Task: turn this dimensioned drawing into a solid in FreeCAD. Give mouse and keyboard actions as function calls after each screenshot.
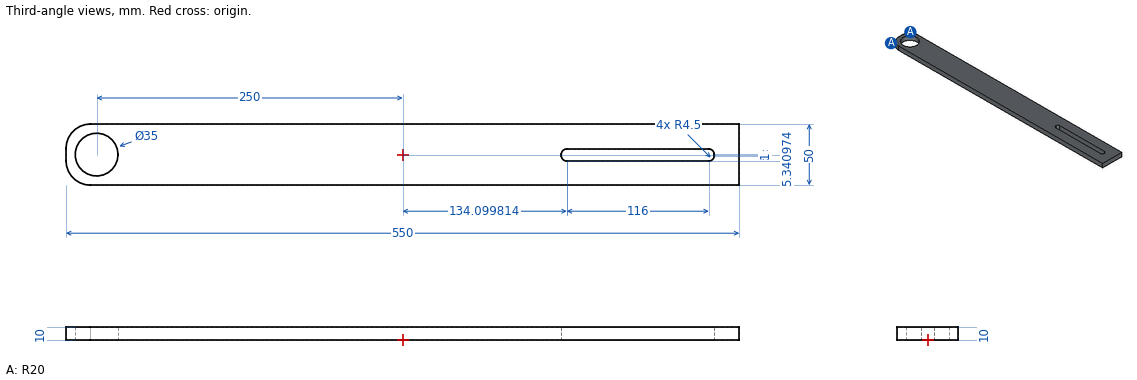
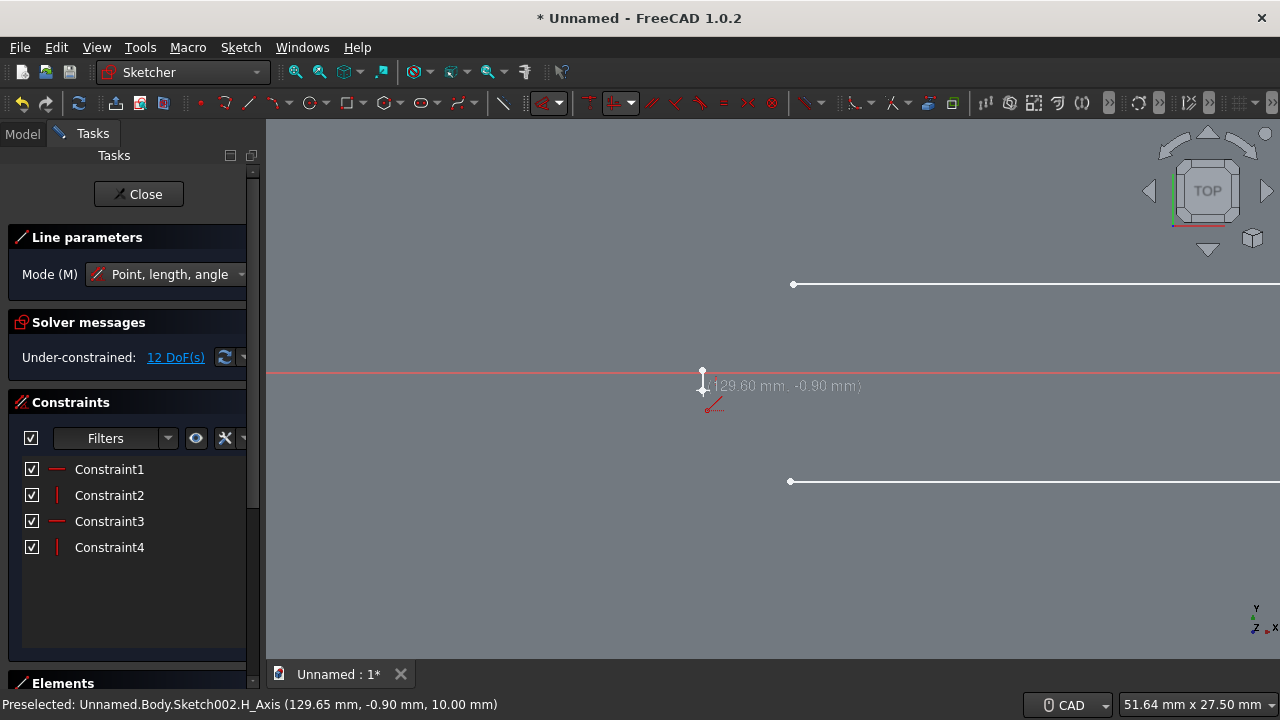
key(g)
key(3)
key(a)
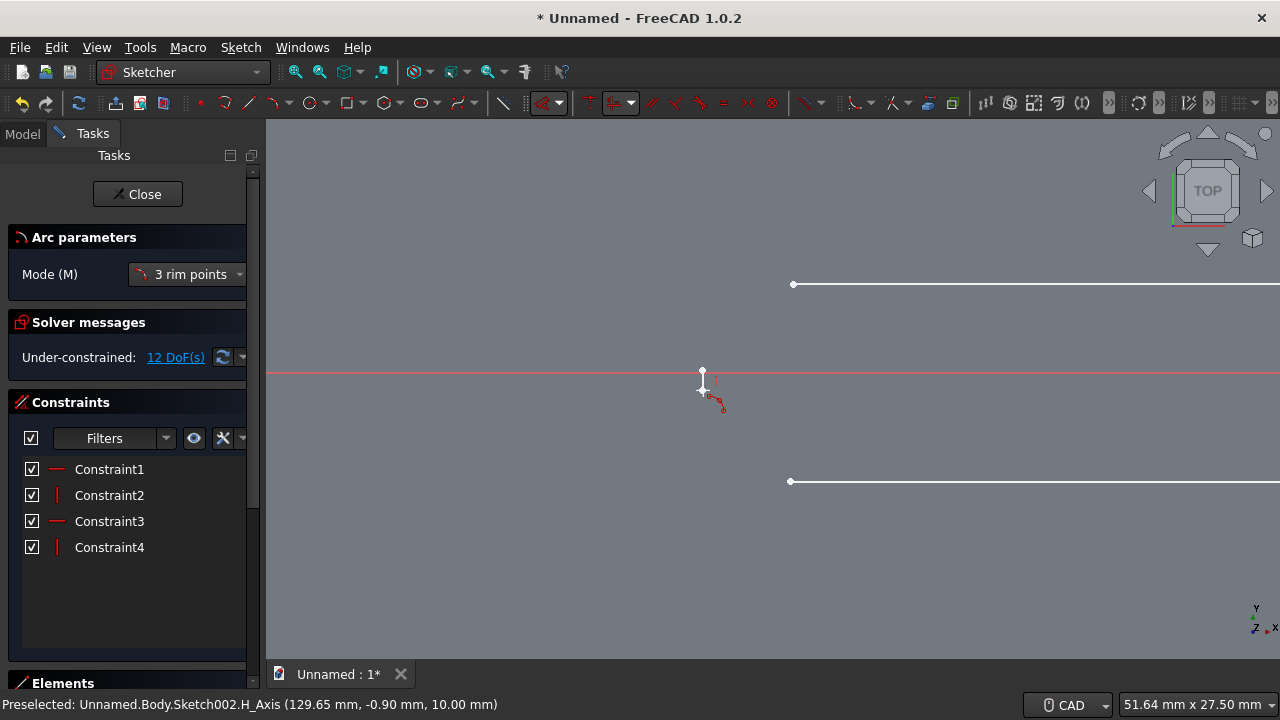
scroll(710, 390, down, 11)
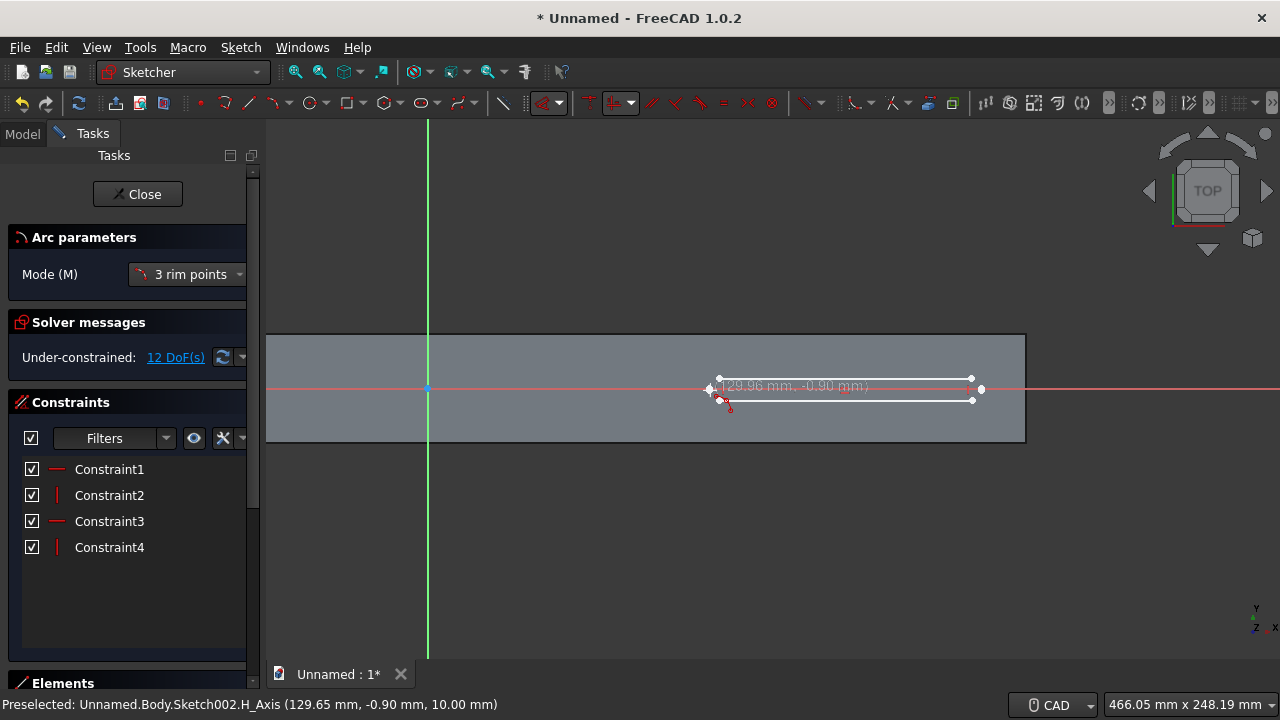
scroll(972, 400, up, 2)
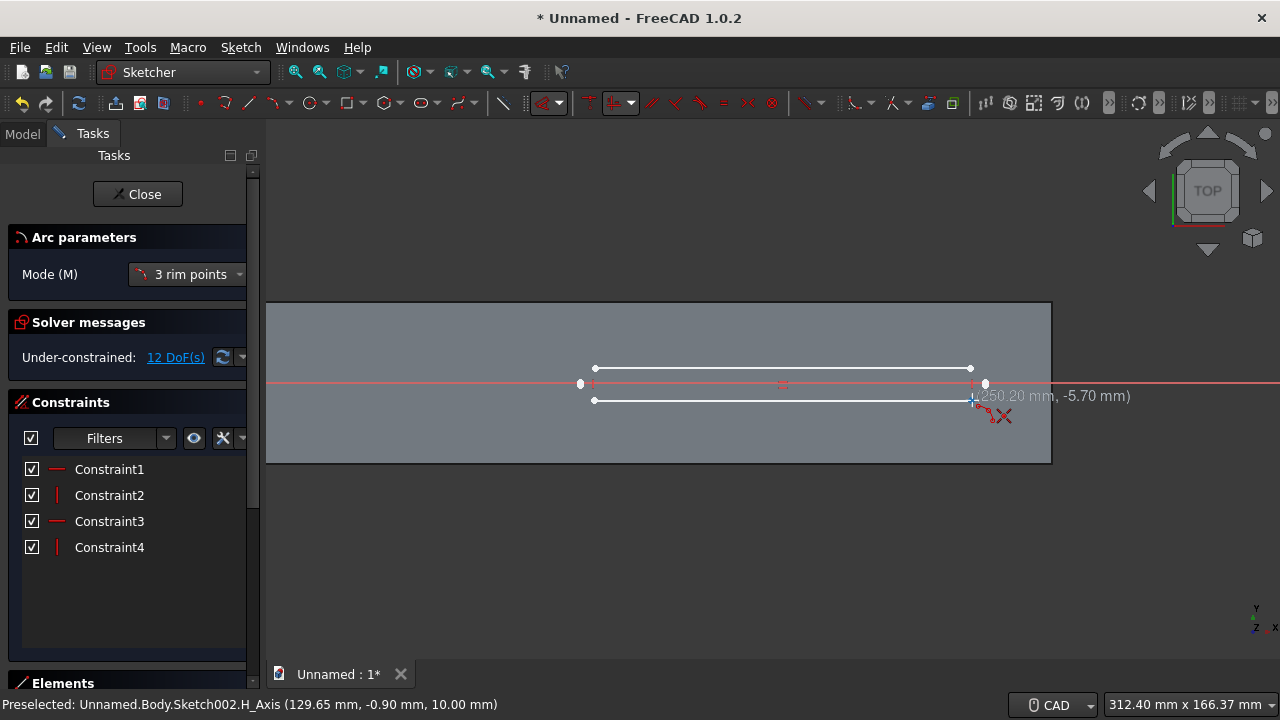
click(972, 401)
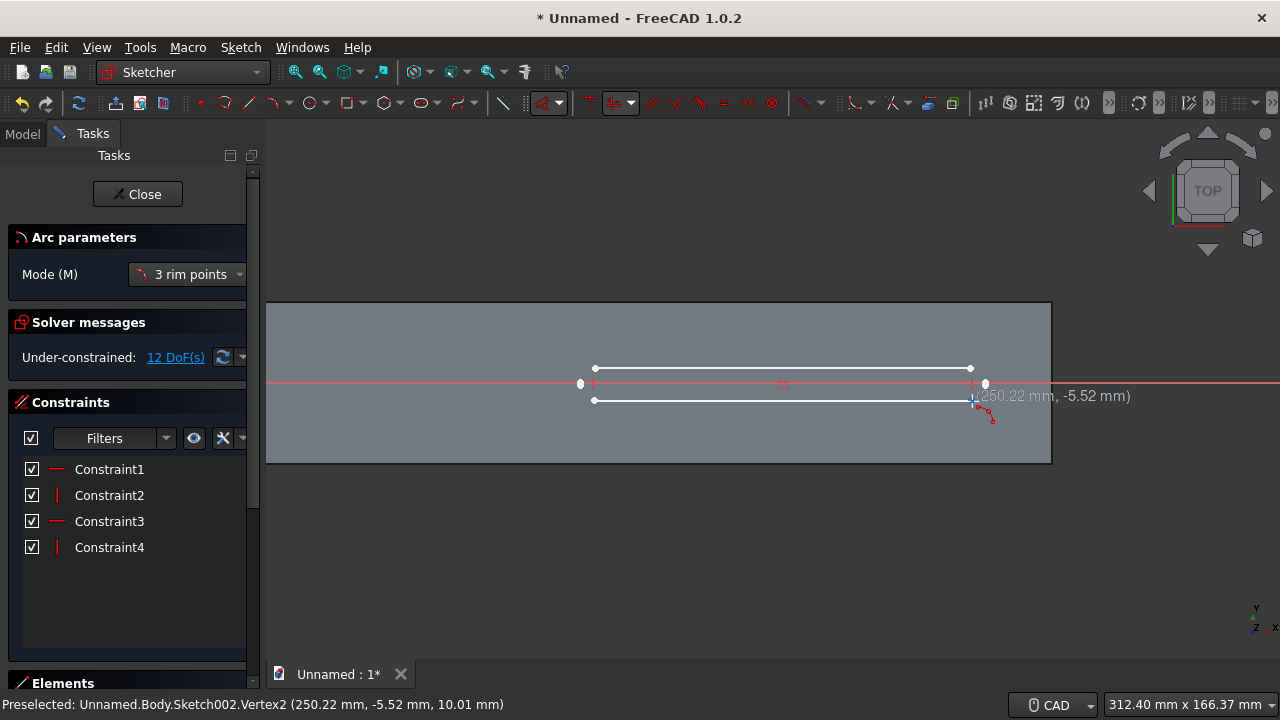
scroll(986, 385, up, 12)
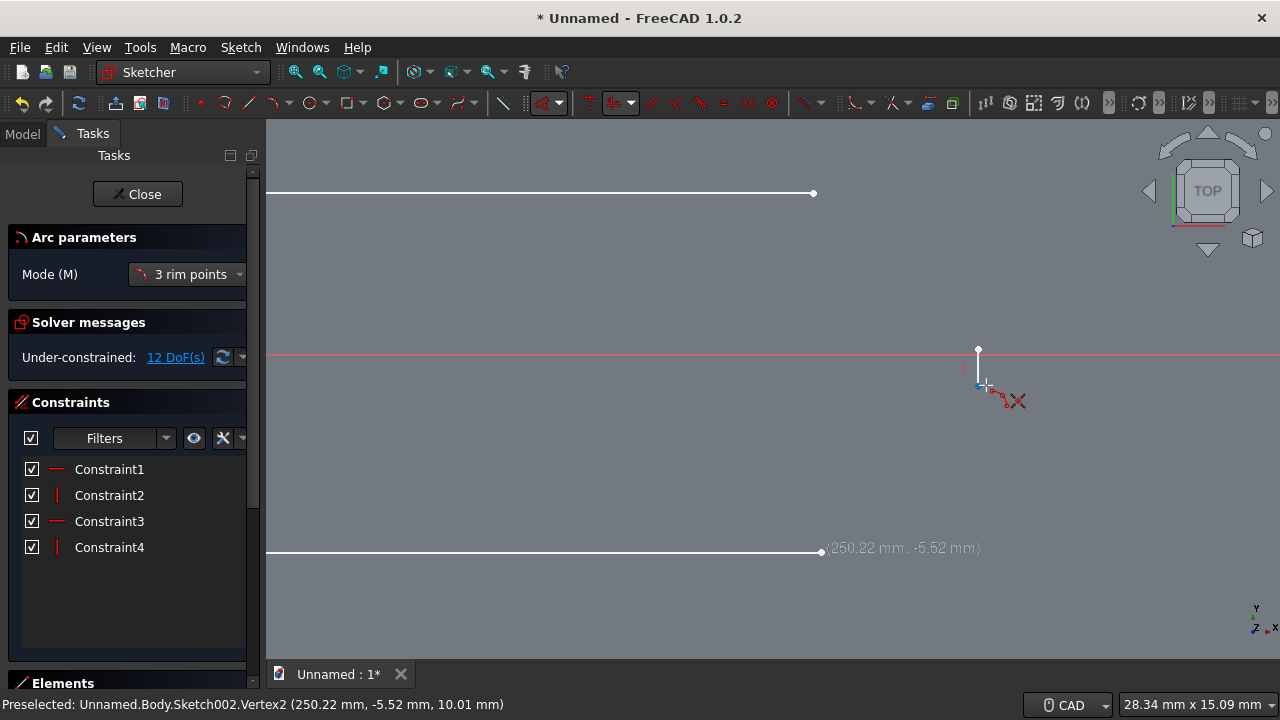
click(978, 386)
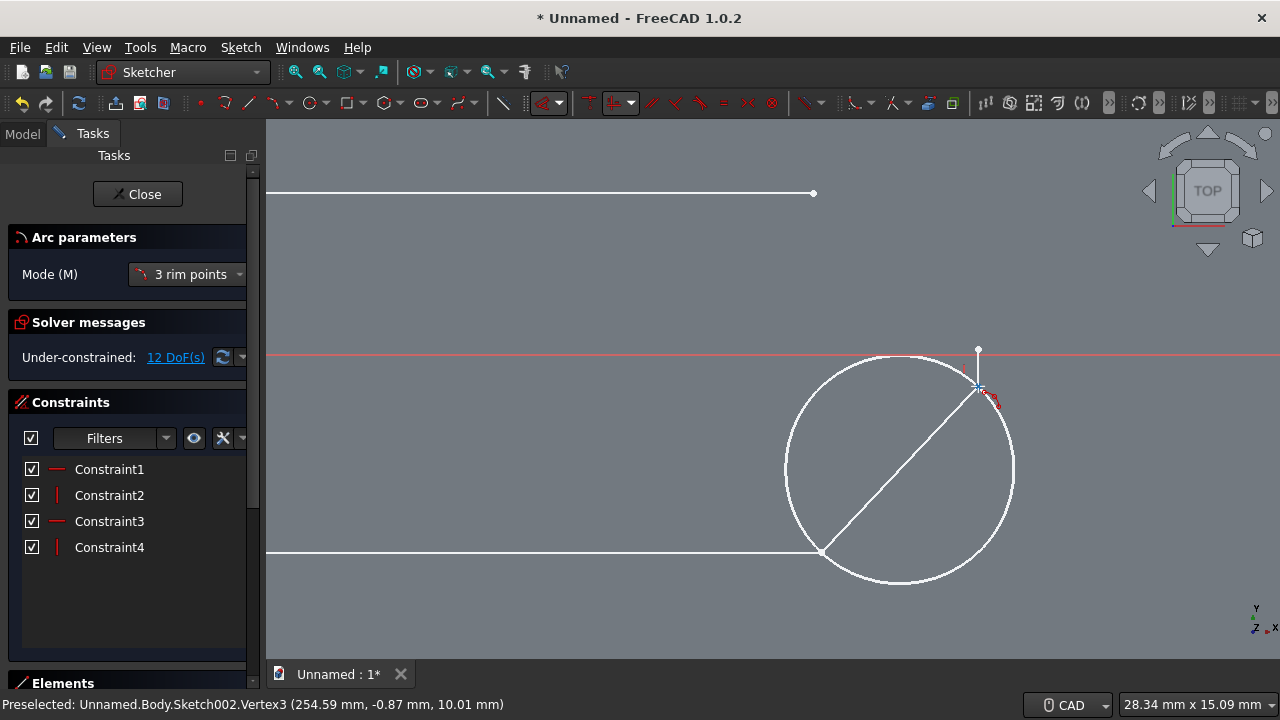
scroll(982, 390, down, 14)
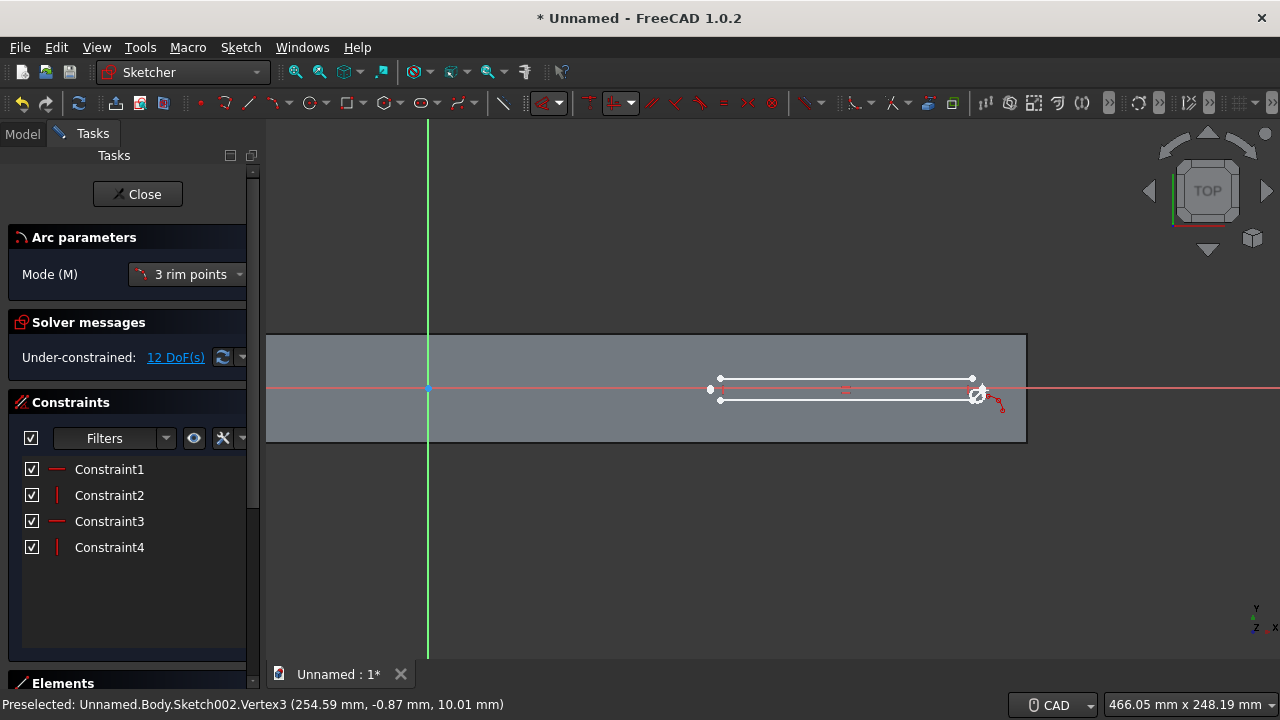
scroll(980, 397, up, 9)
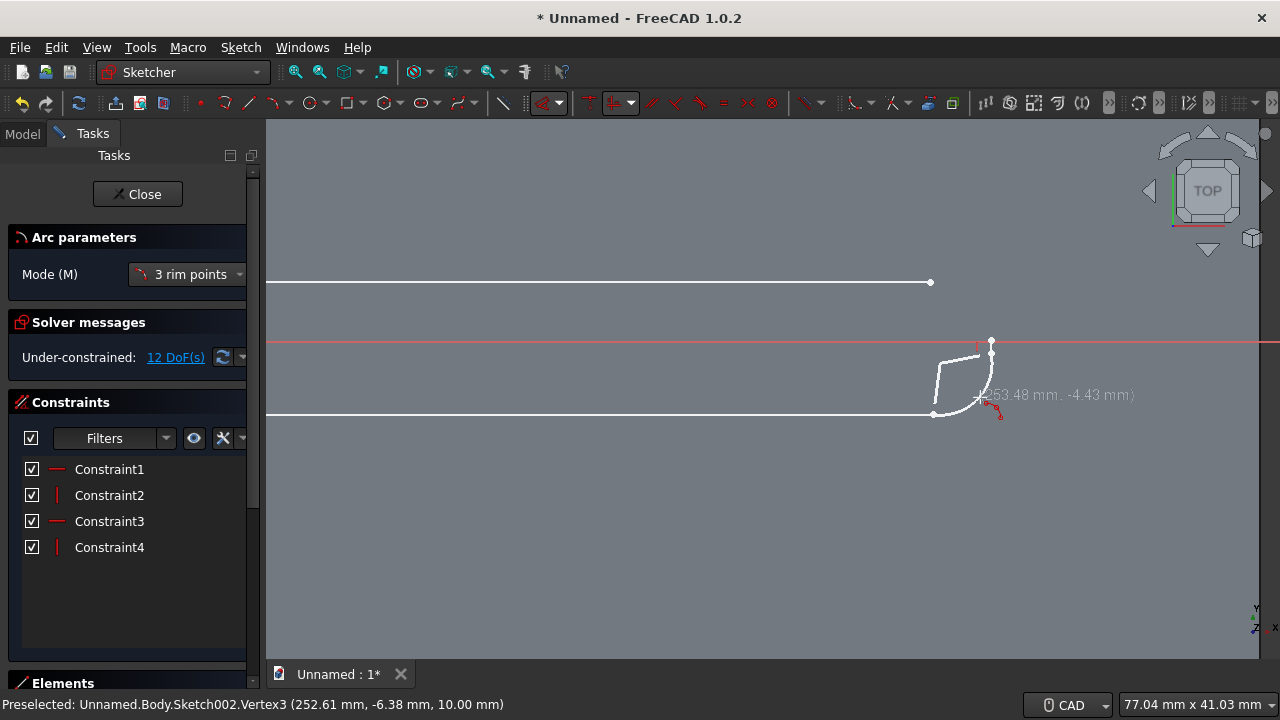
click(974, 395)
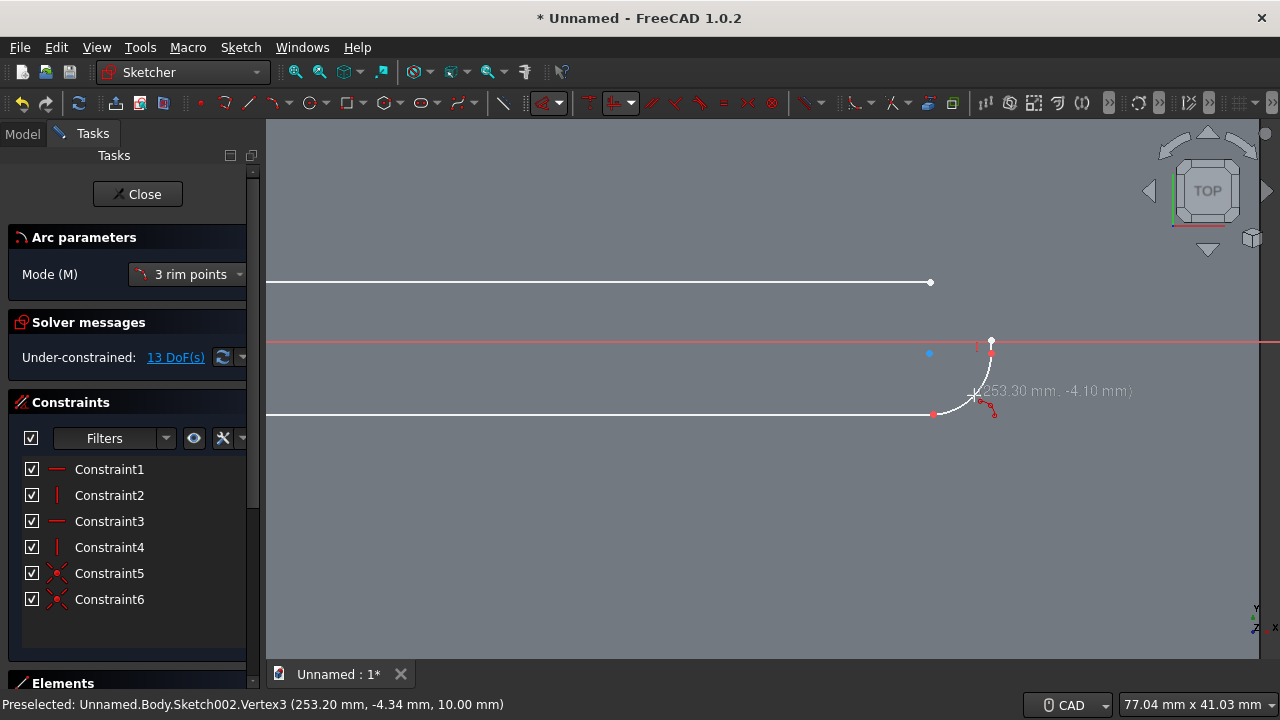
scroll(991, 340, up, 11)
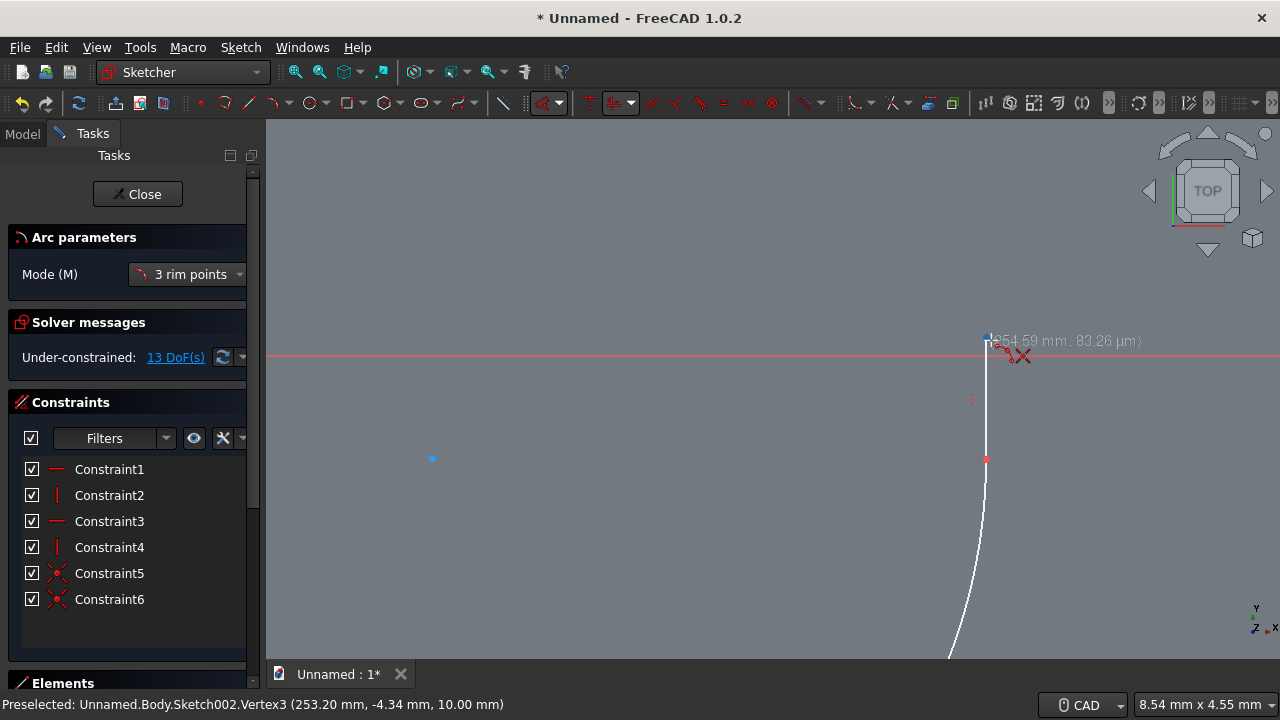
click(986, 338)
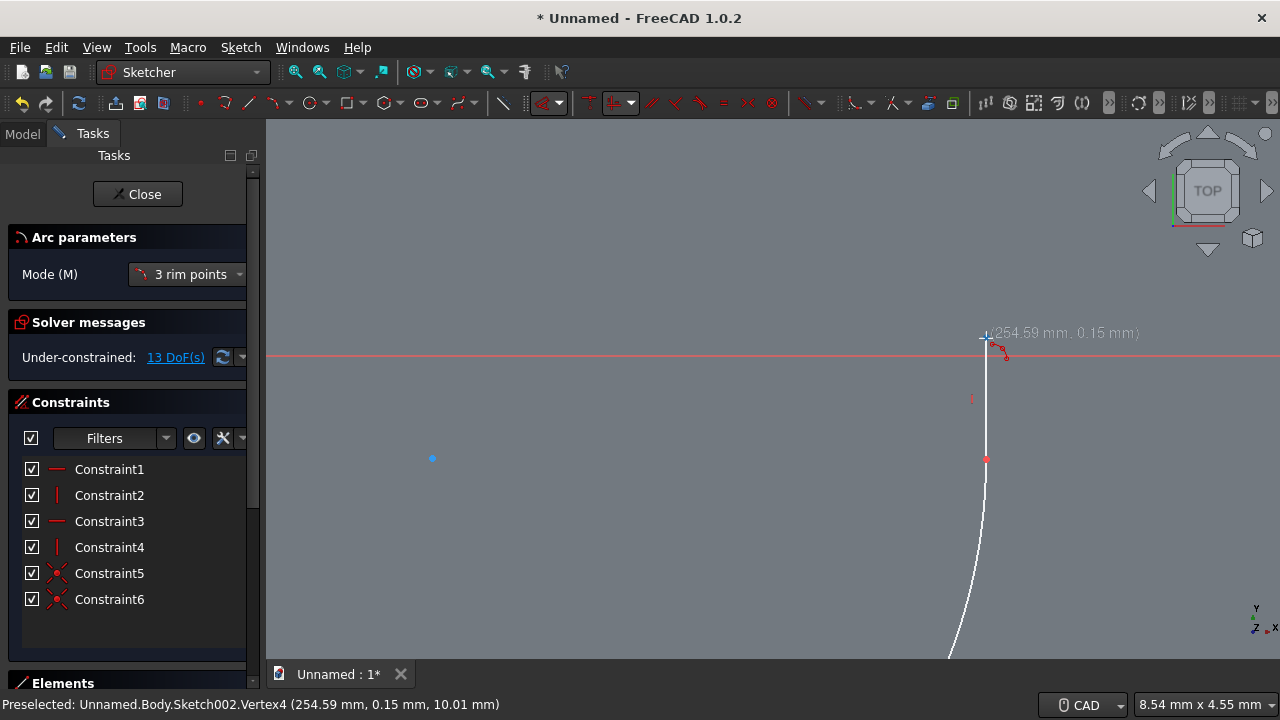
scroll(704, 389, down, 15)